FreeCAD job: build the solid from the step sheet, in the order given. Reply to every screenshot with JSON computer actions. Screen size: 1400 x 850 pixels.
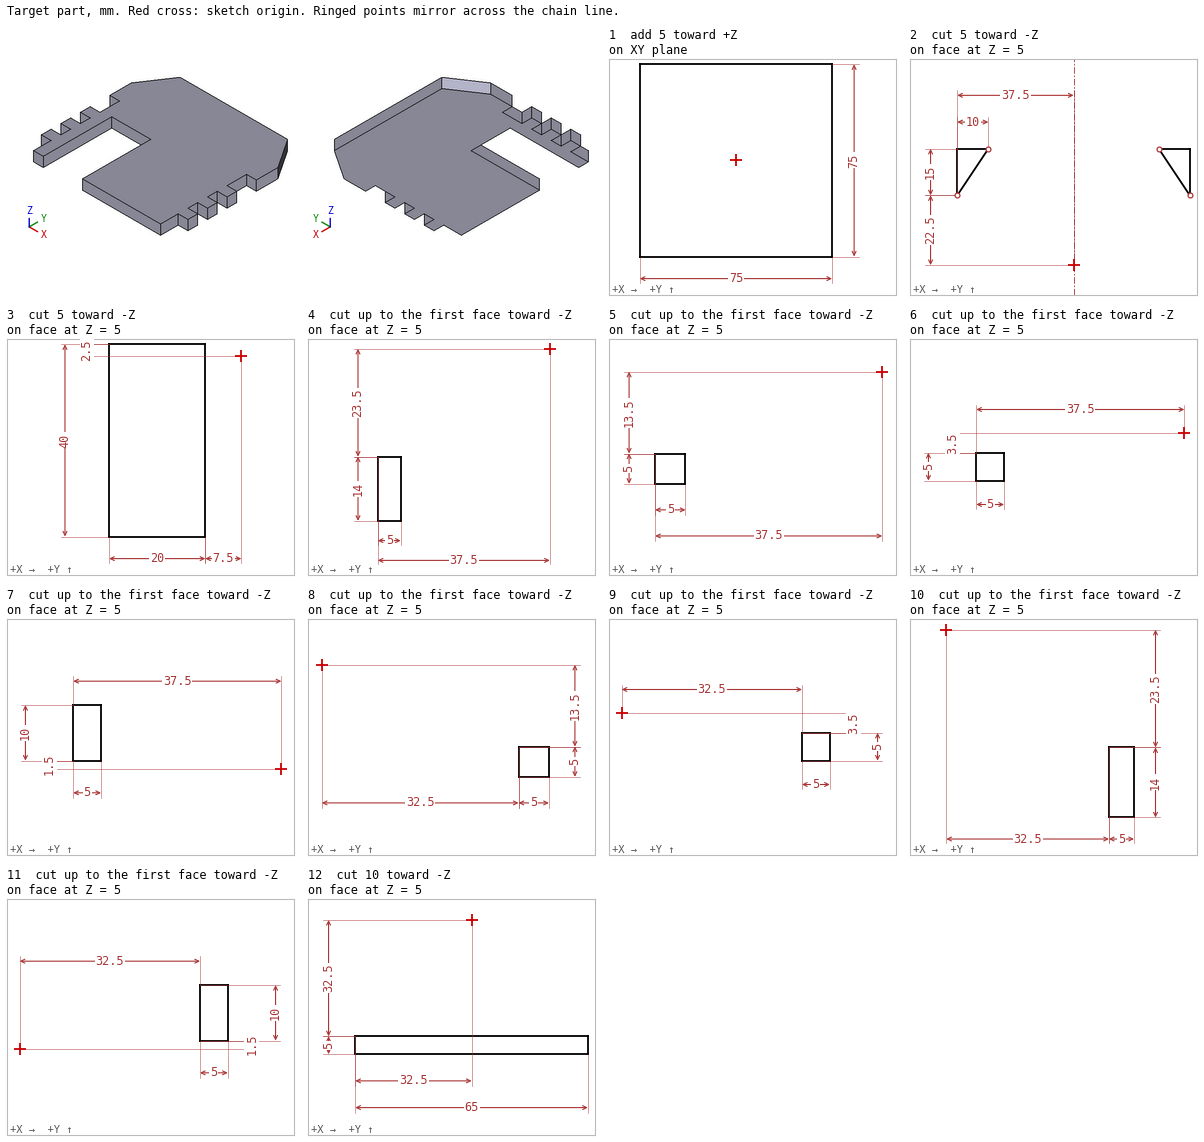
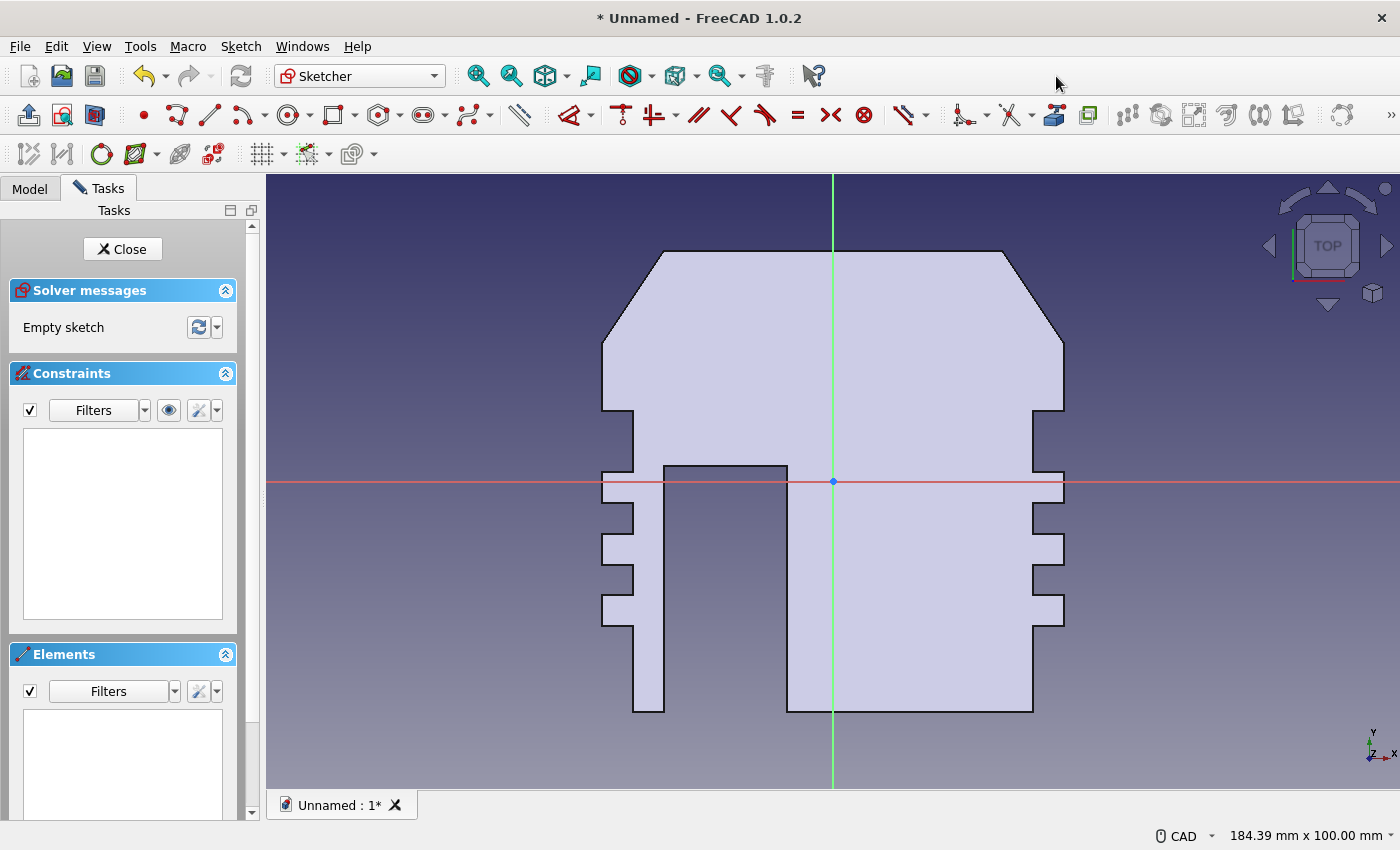
{"action": "scroll", "coordinate": [916, 737], "scroll_direction": "up", "scroll_amount": 3}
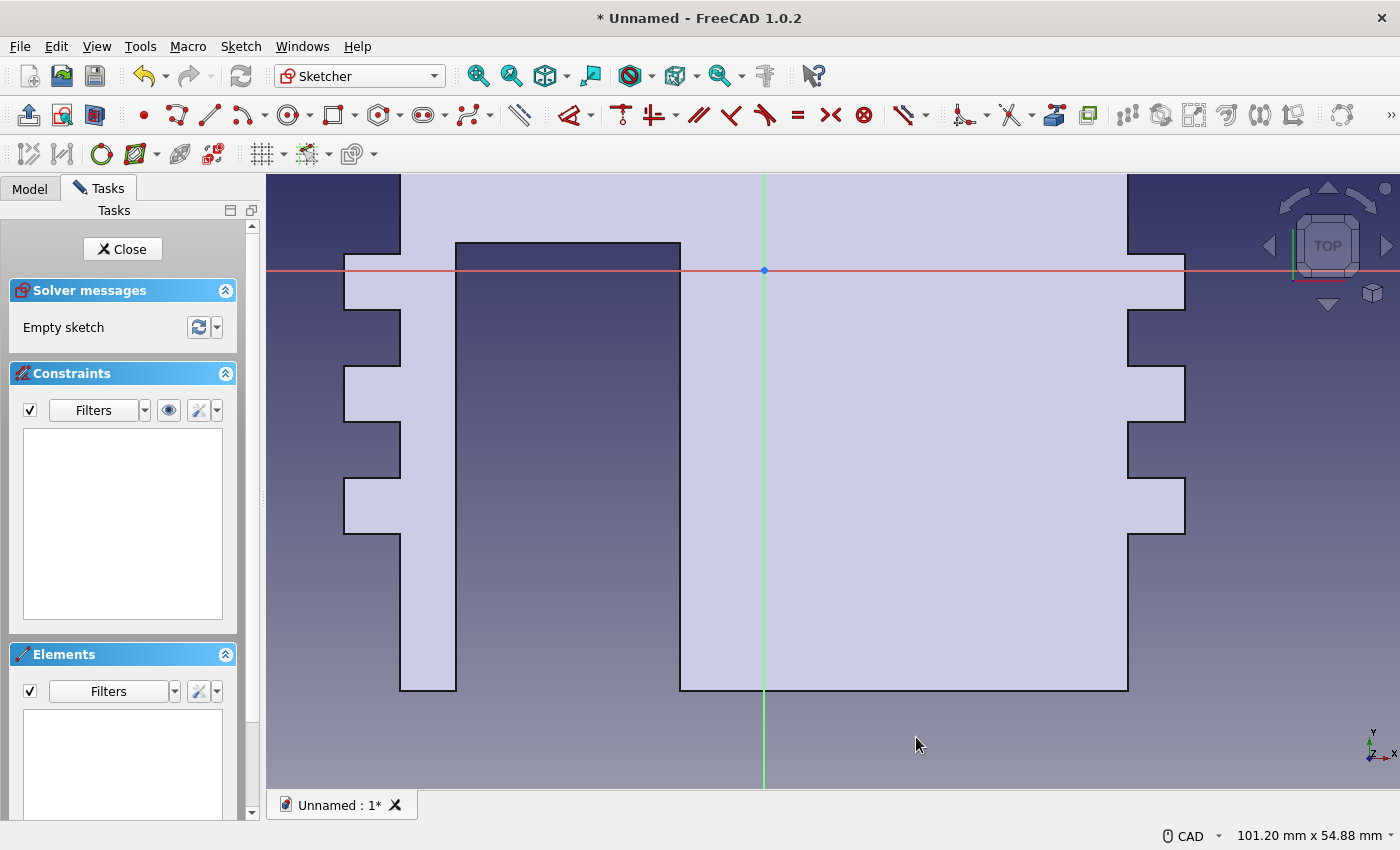
{"action": "left_click", "coordinate": [332, 116]}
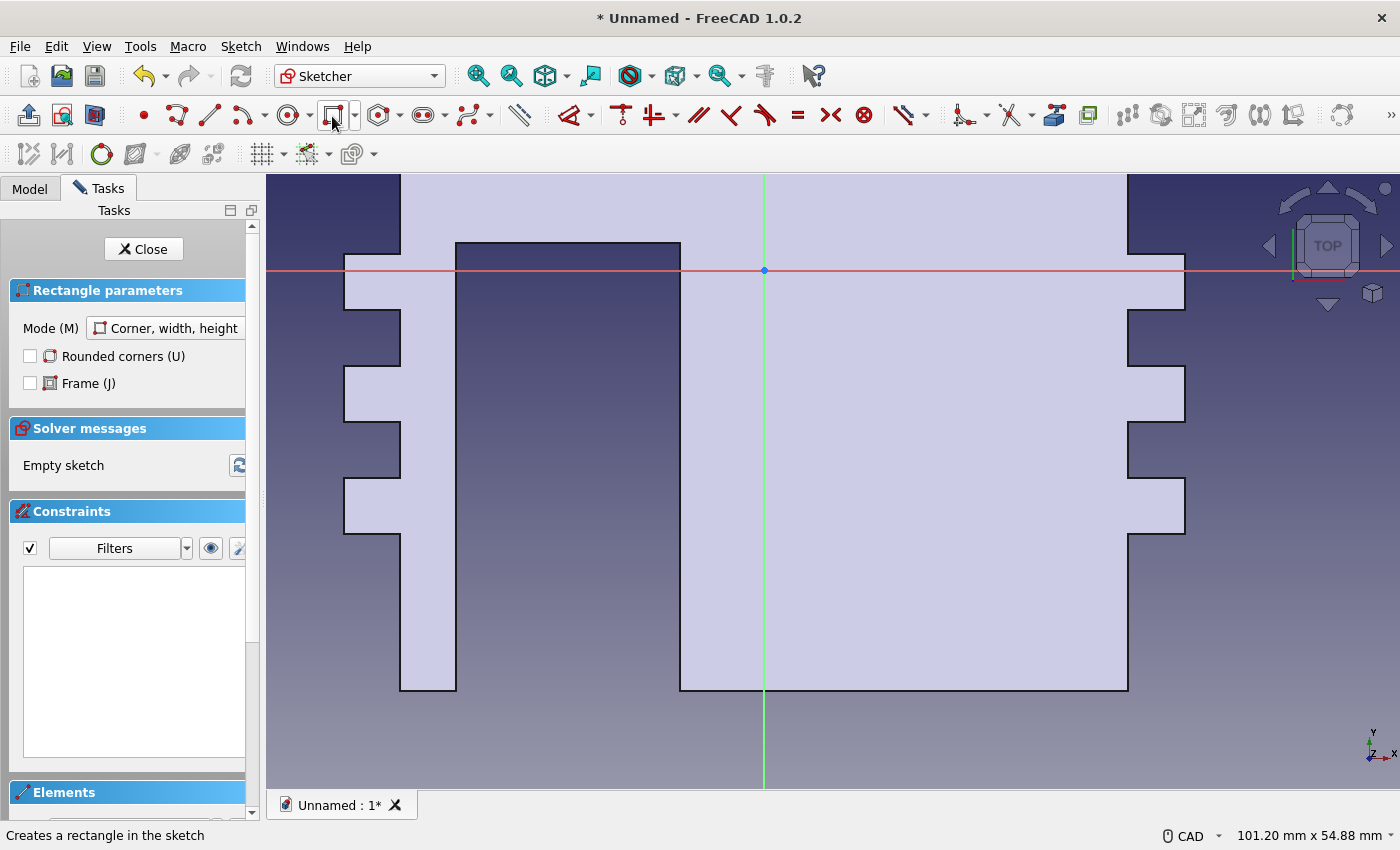
{"action": "left_click", "coordinate": [400, 635]}
{"action": "left_click", "coordinate": [1128, 691]}
{"action": "key", "text": "Escape"}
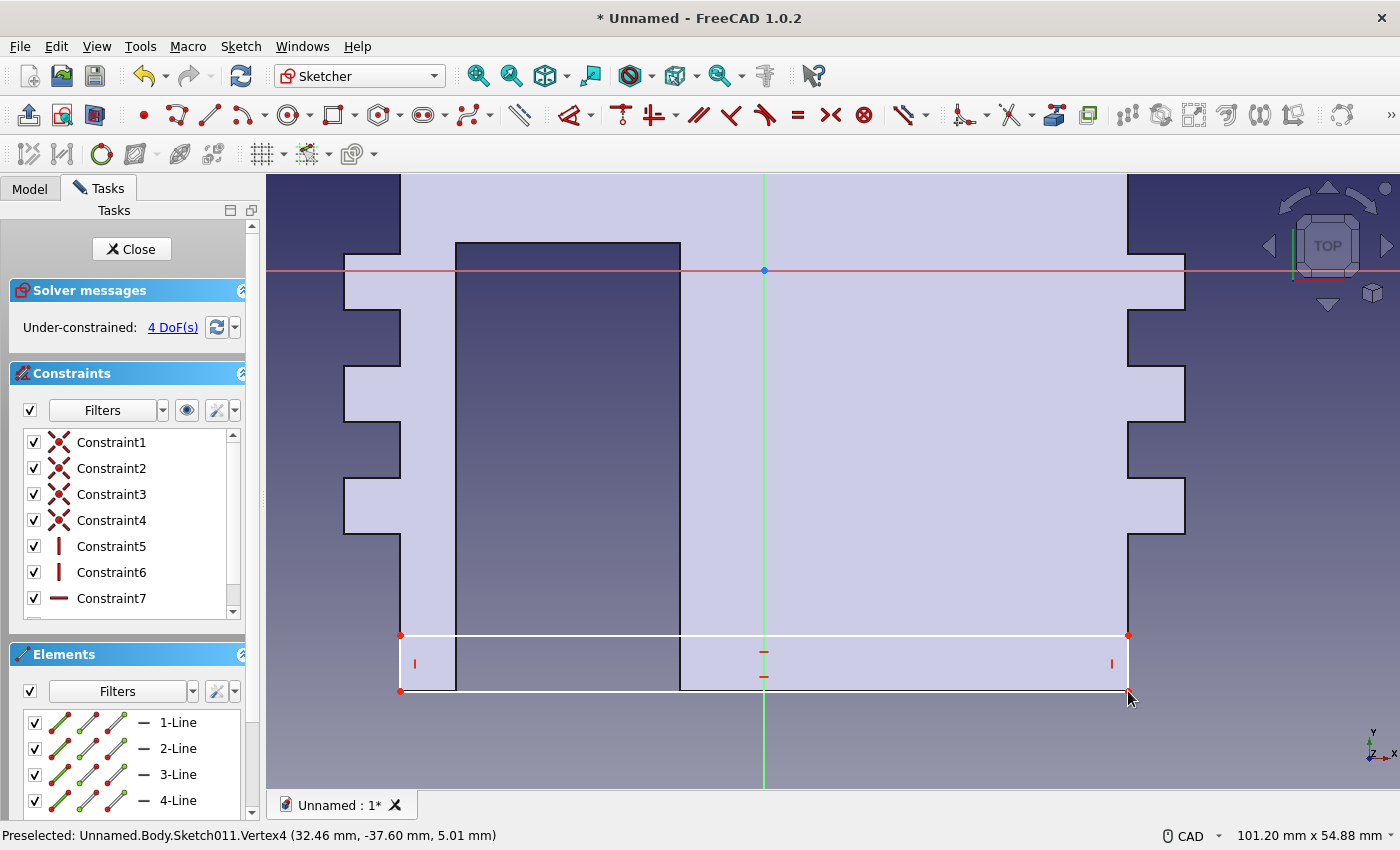
{"action": "left_click", "coordinate": [568, 116]}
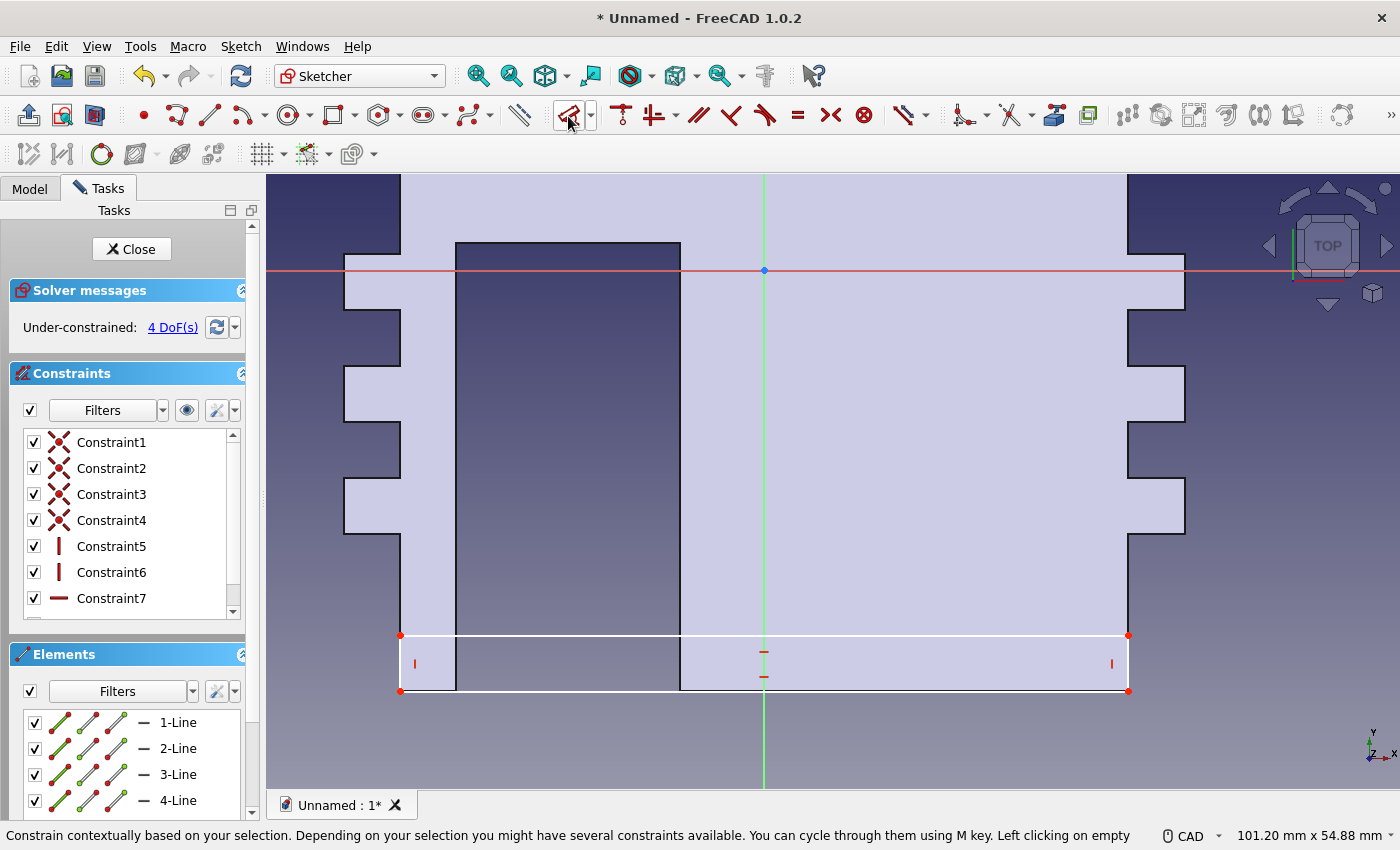
{"action": "left_click", "coordinate": [400, 653]}
{"action": "left_click", "coordinate": [366, 664]}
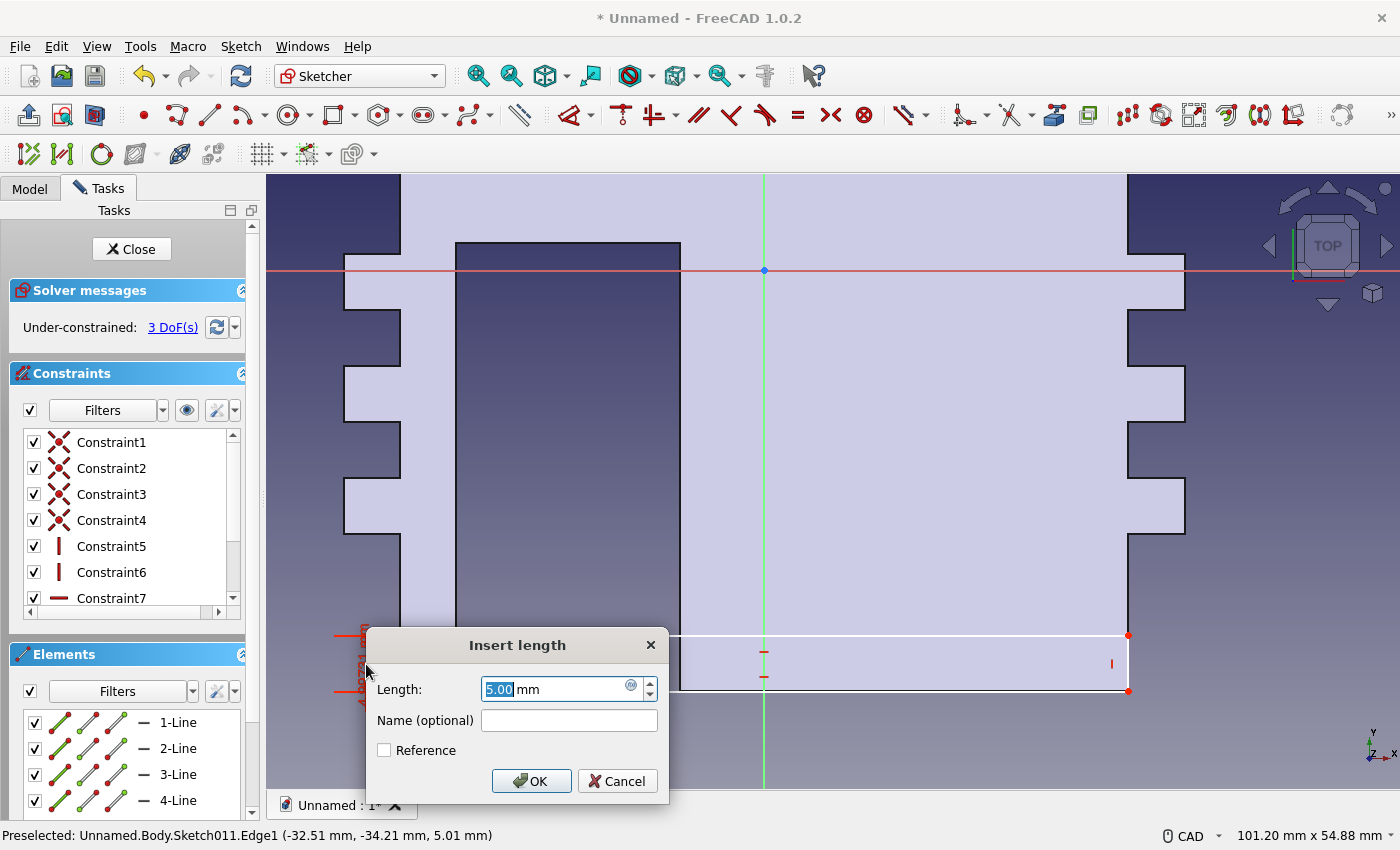
{"action": "type", "text": "5"}
{"action": "key", "text": "Return"}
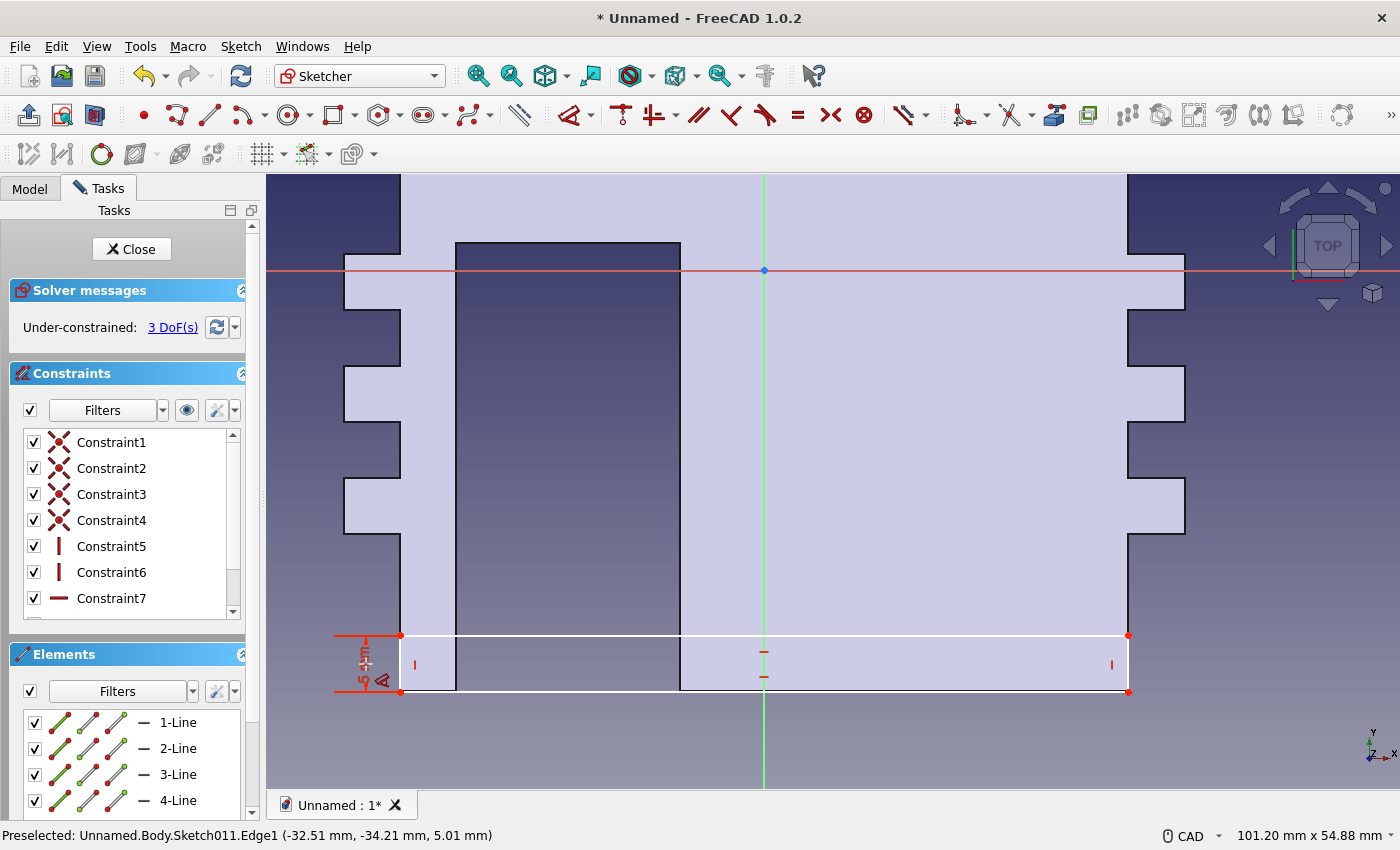
{"action": "left_click", "coordinate": [618, 692]}
{"action": "left_click", "coordinate": [597, 726]}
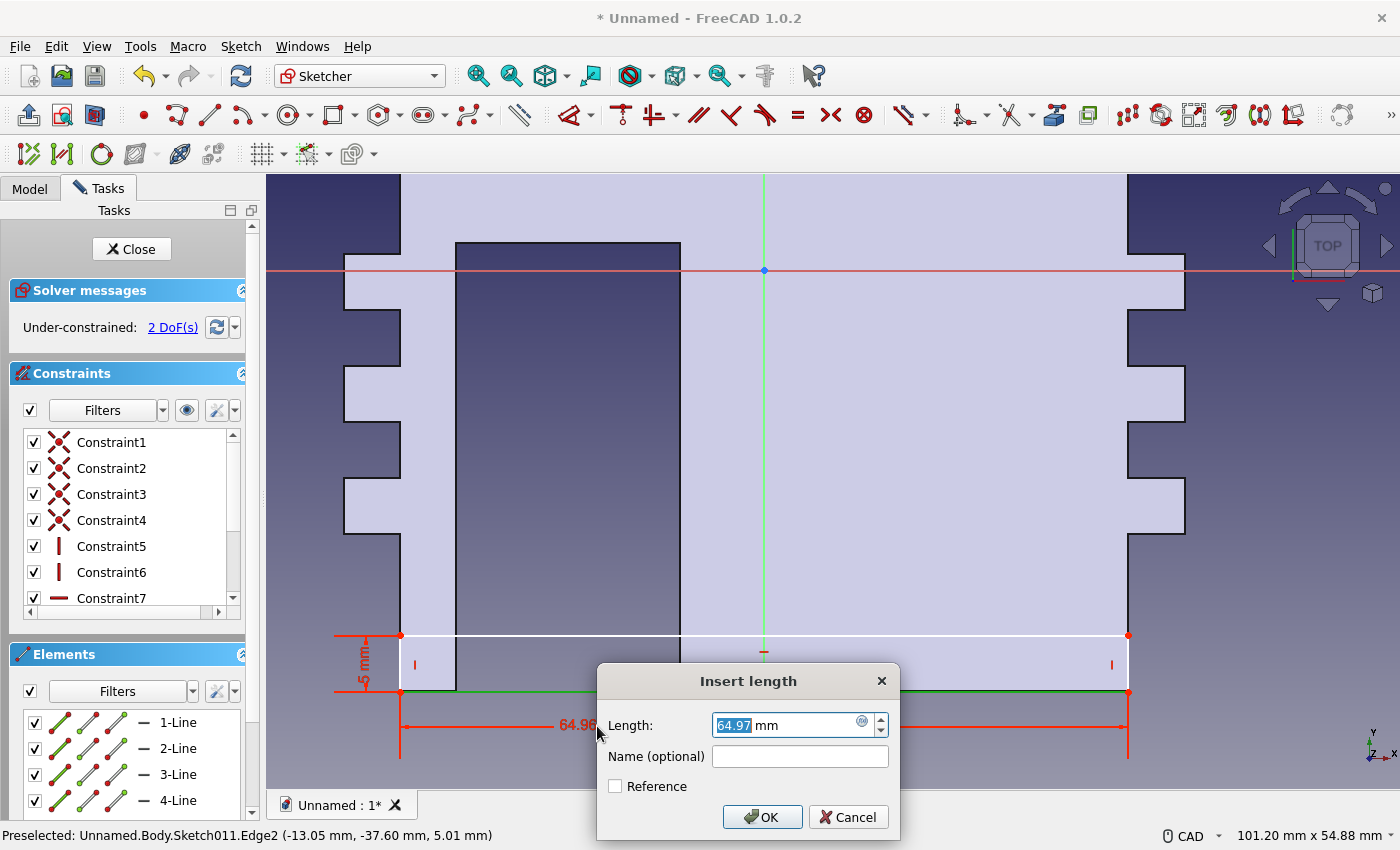
{"action": "type", "text": "65"}
{"action": "key", "text": "Return"}